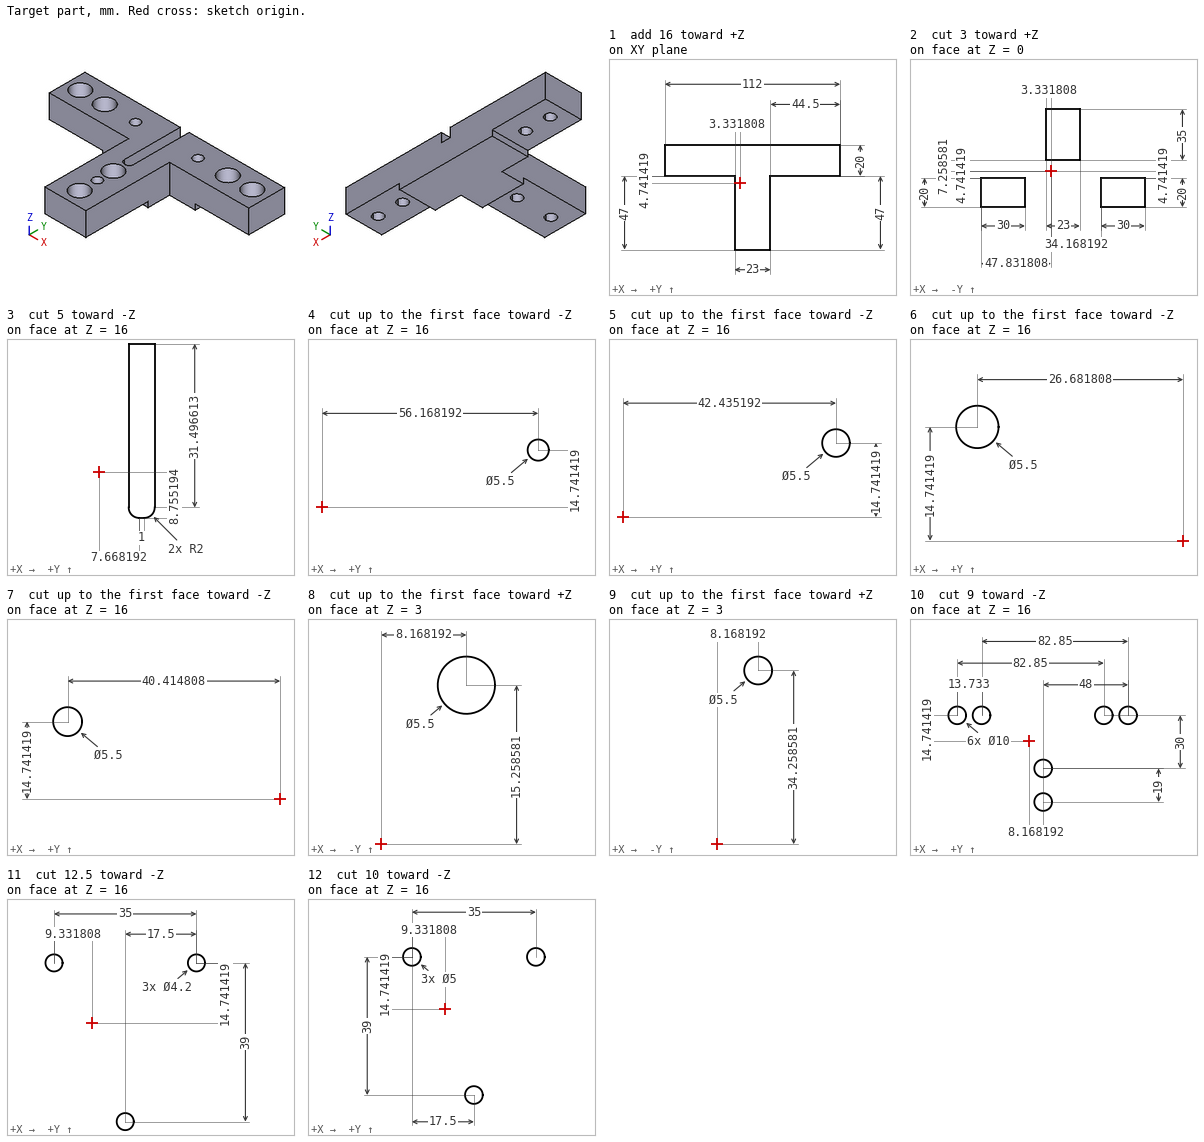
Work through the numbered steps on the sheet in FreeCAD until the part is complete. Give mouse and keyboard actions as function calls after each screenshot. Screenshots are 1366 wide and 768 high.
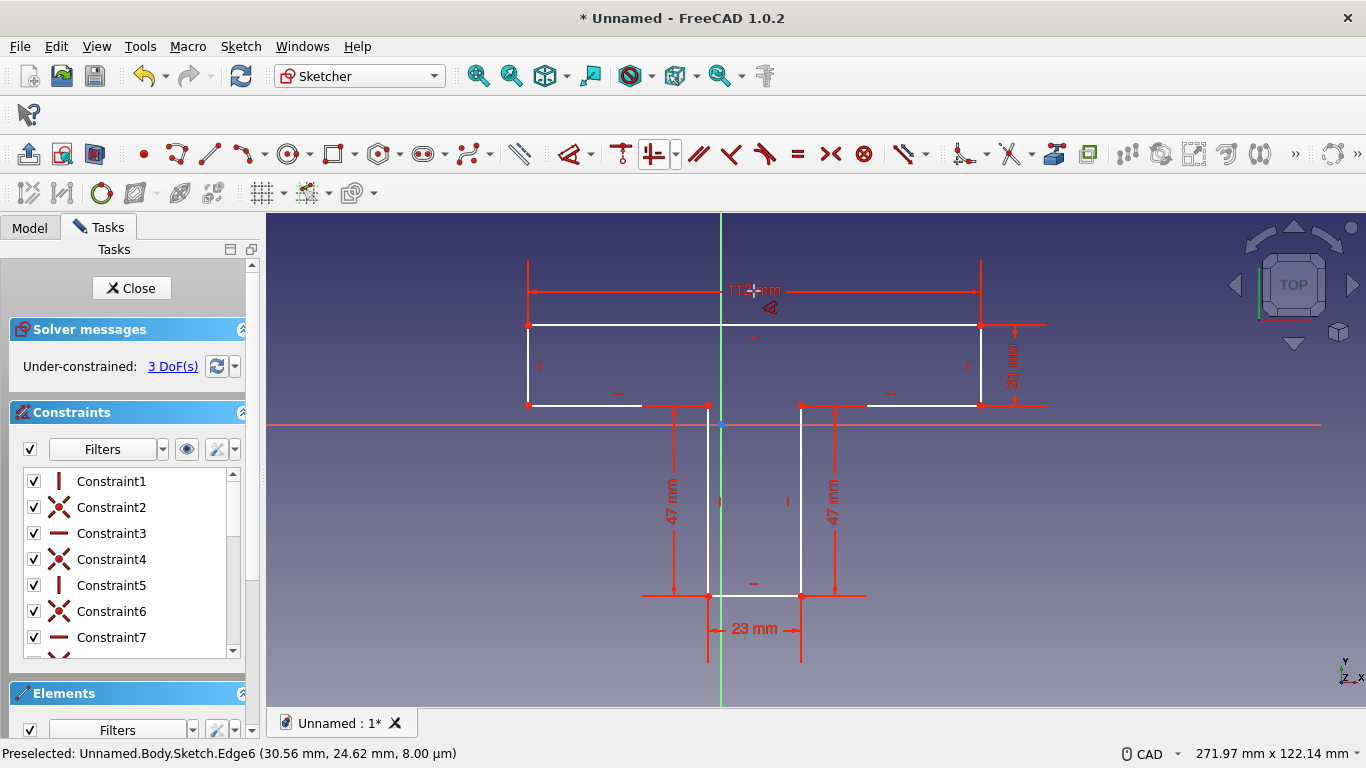
click(855, 406)
click(891, 372)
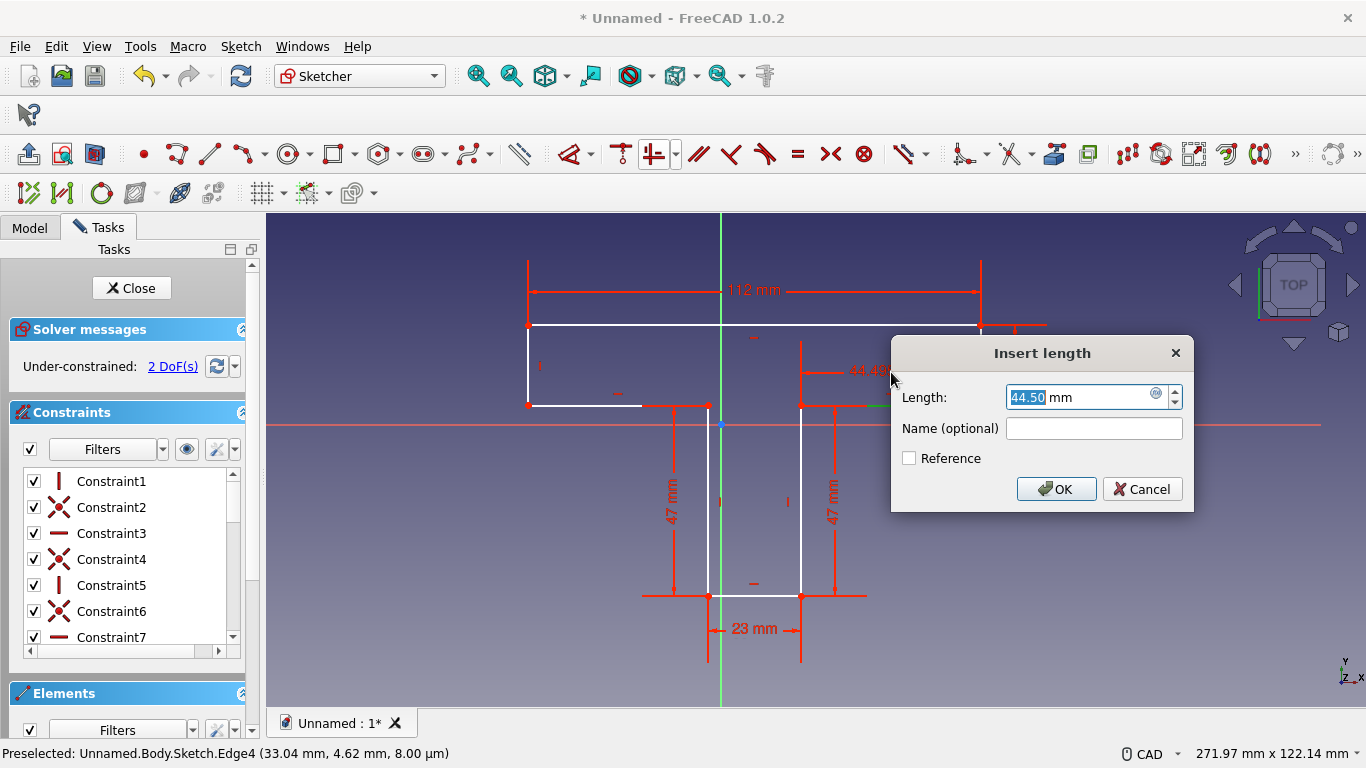
text(44.5)
key(Return)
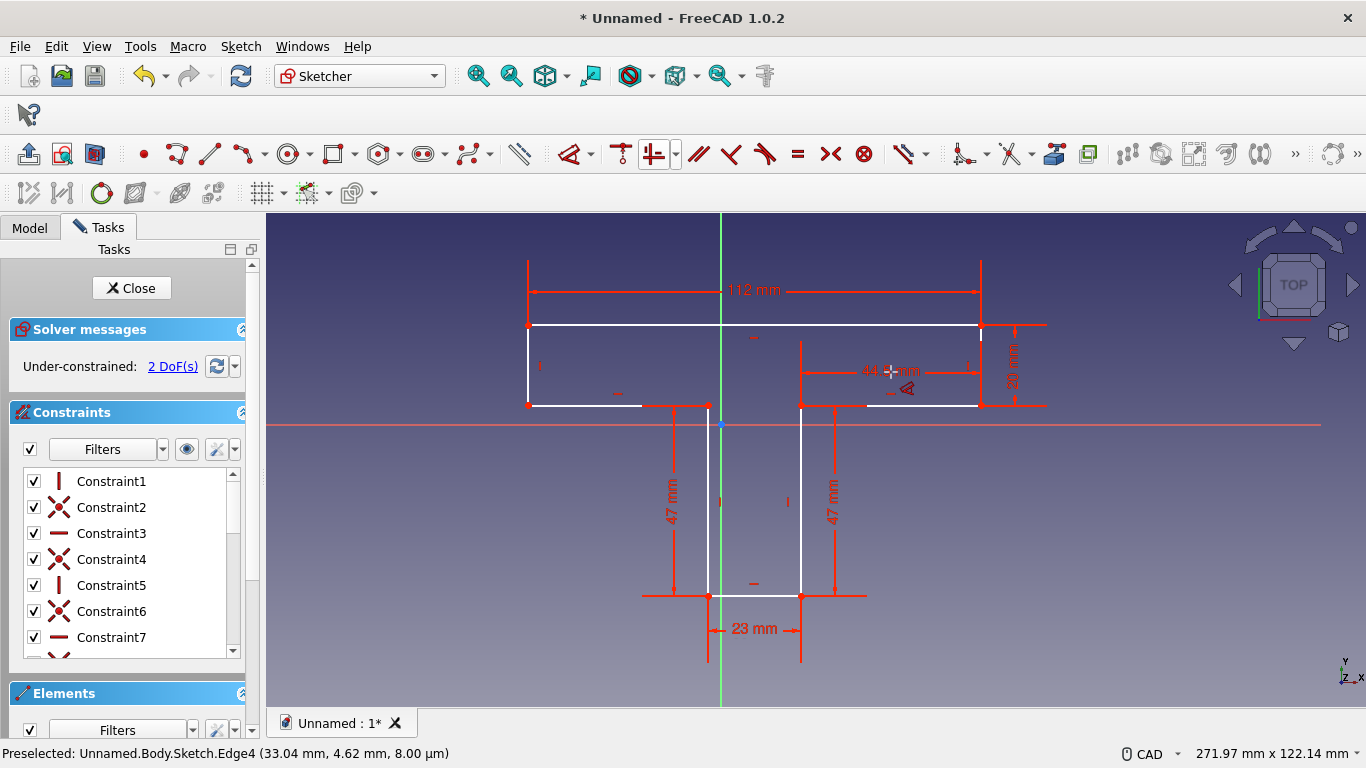
scroll(708, 406, up, 6)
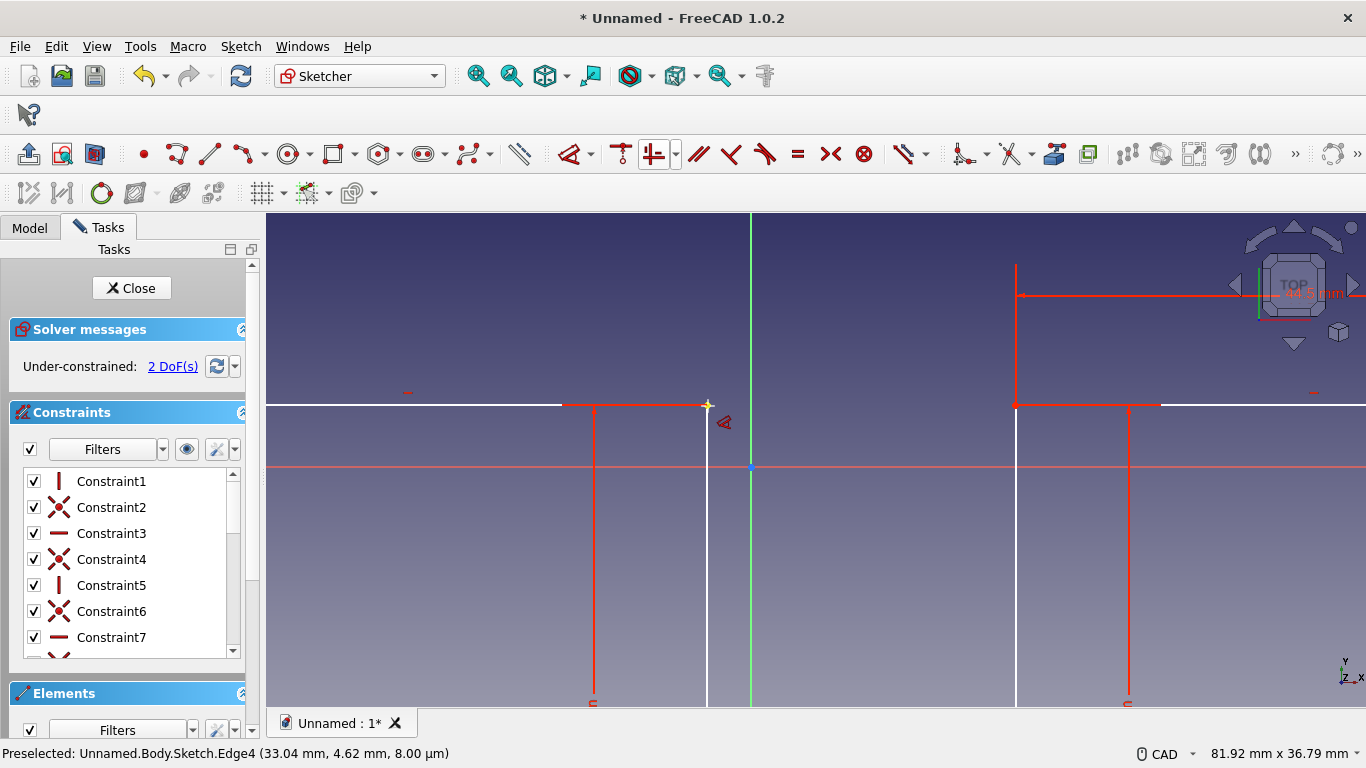
click(707, 405)
click(729, 371)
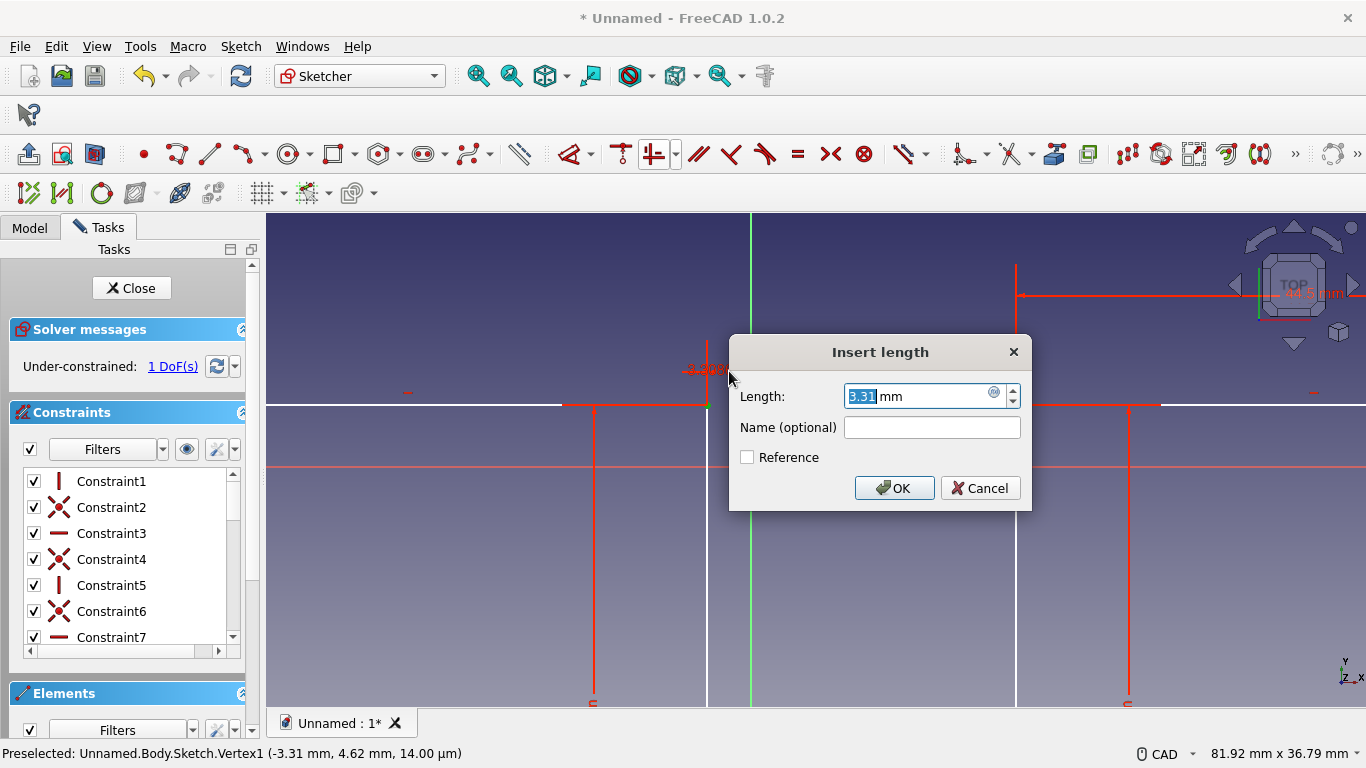
text(3.331808)
key(Return)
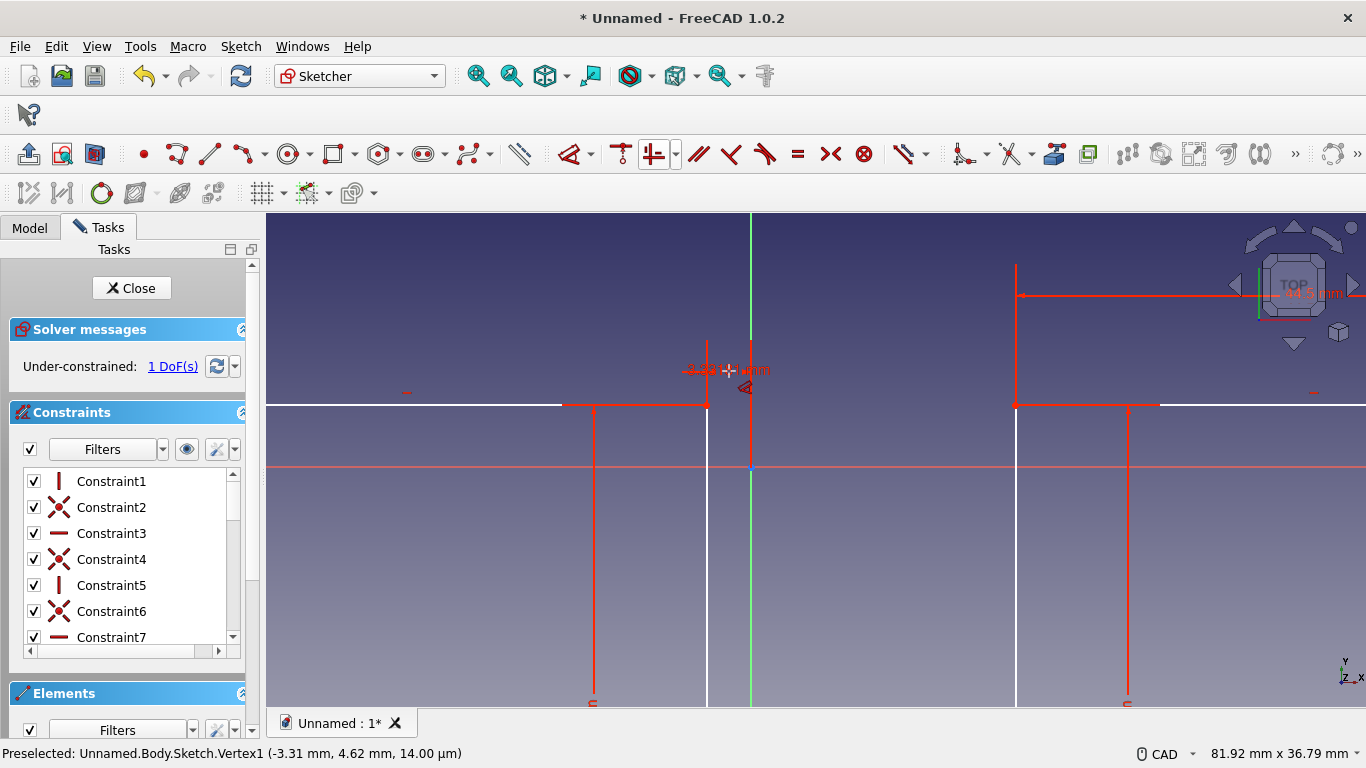
click(707, 405)
click(673, 436)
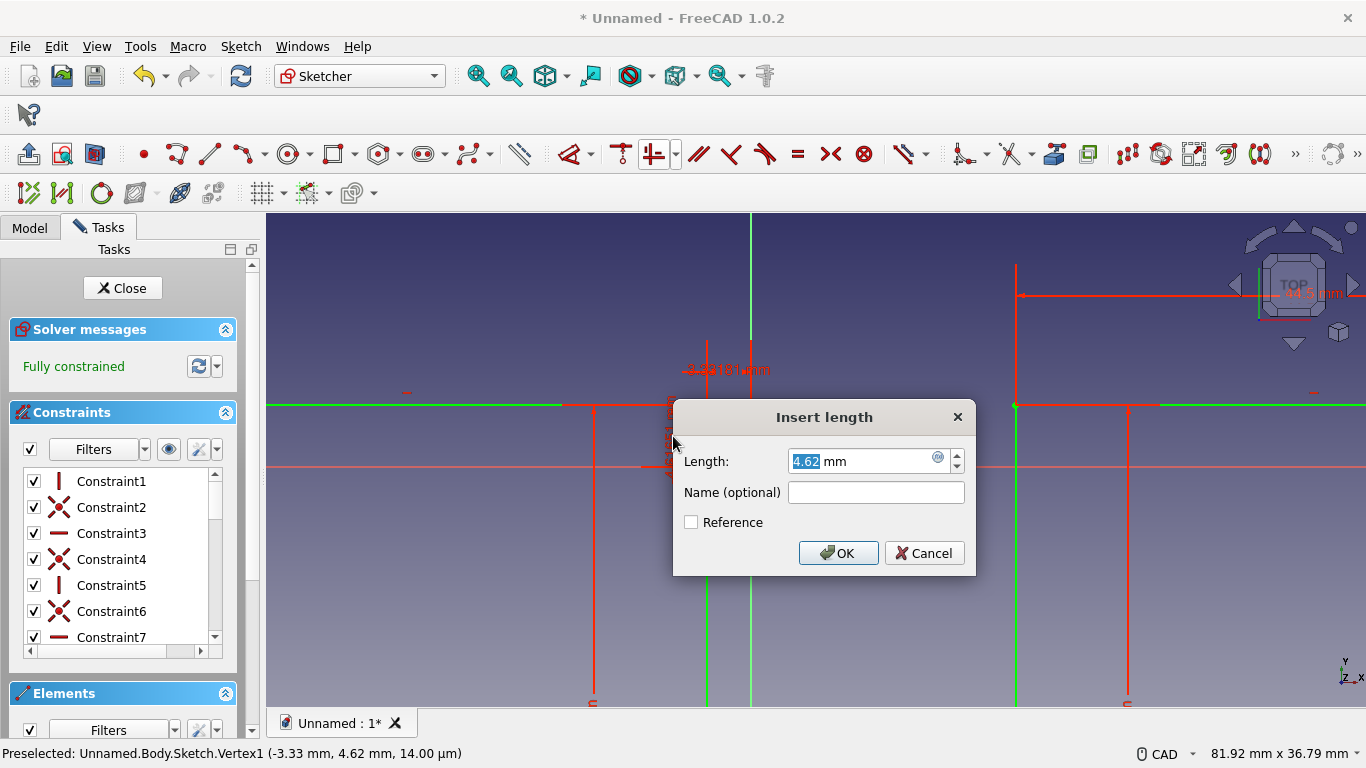
text(4.741419)
key(Return)
key(Escape)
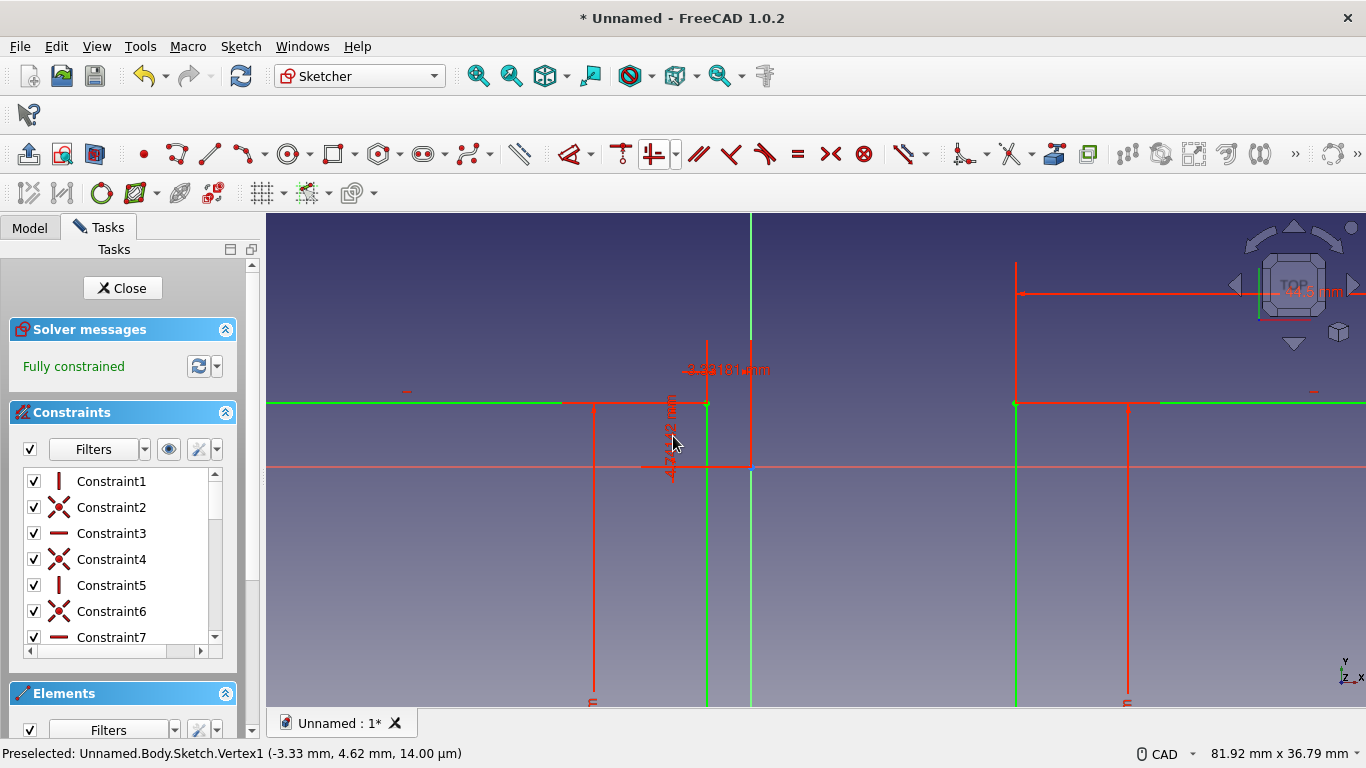
click(123, 288)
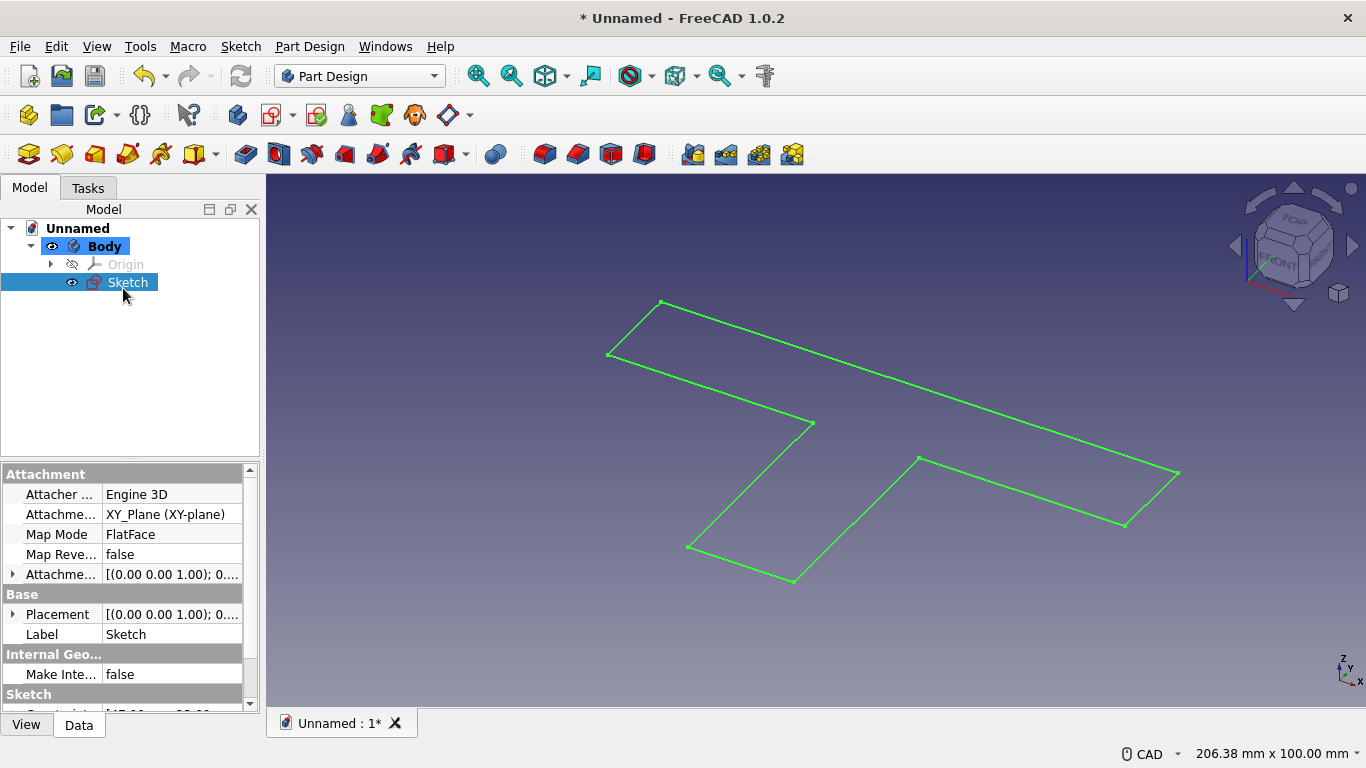
click(29, 154)